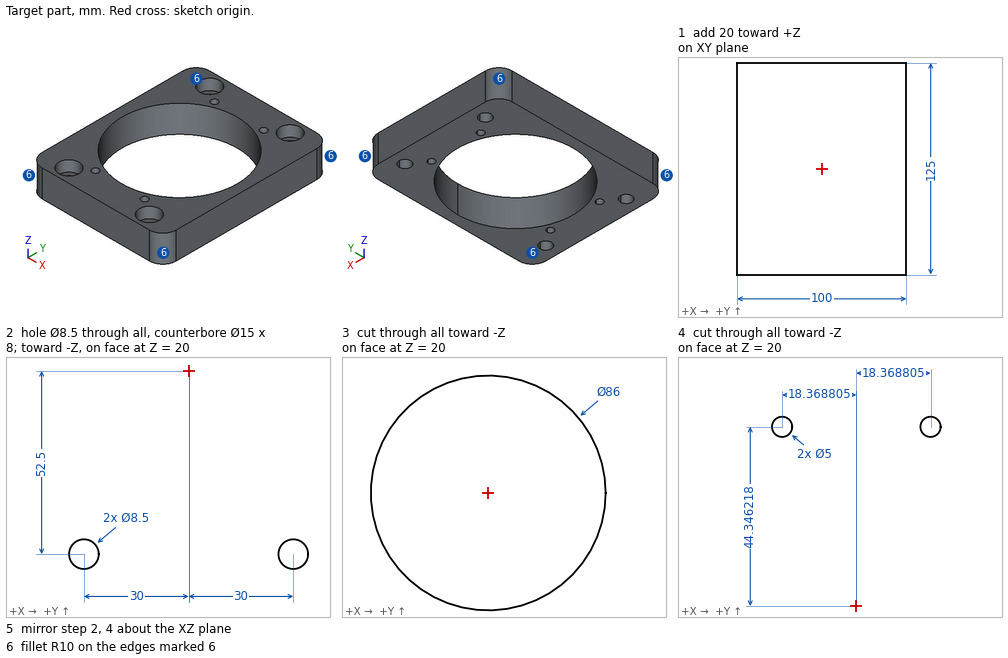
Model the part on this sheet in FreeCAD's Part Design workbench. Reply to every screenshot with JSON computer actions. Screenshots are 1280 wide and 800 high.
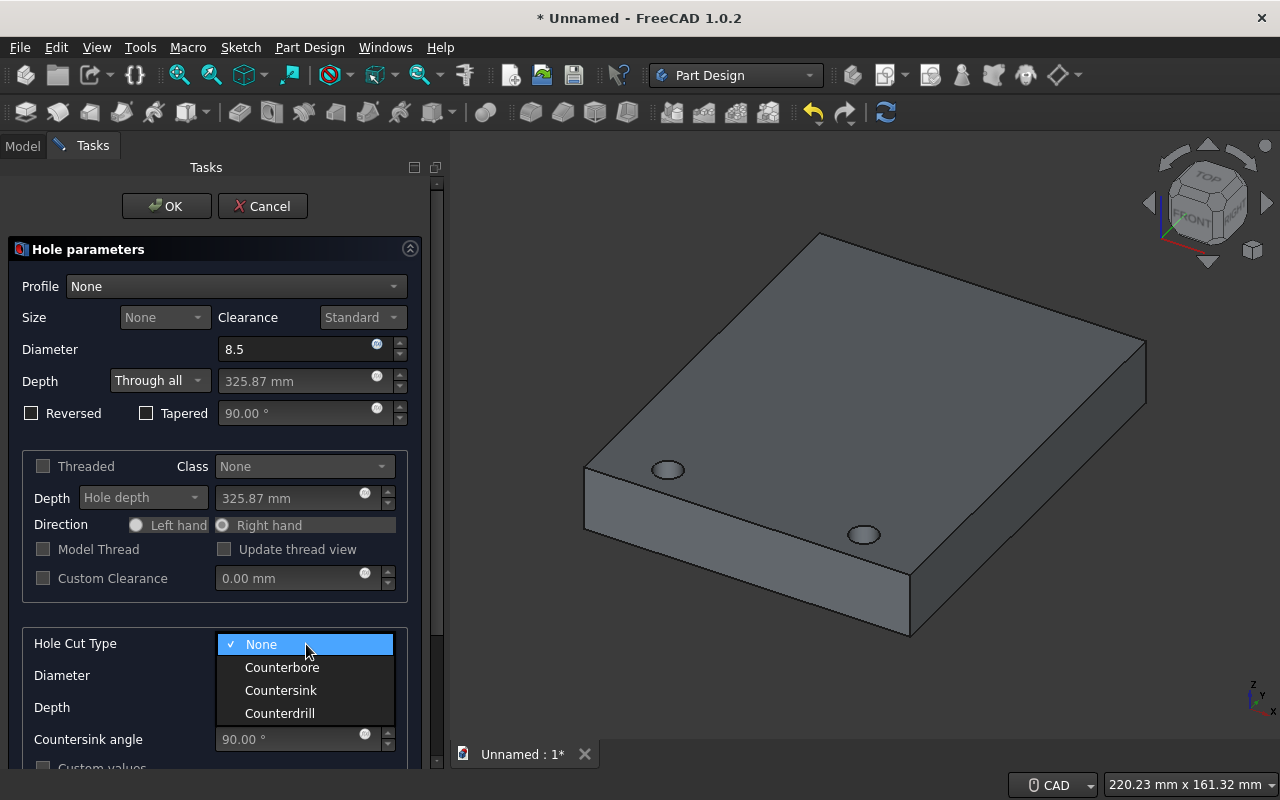
{"action": "left_click", "coordinate": [304, 668]}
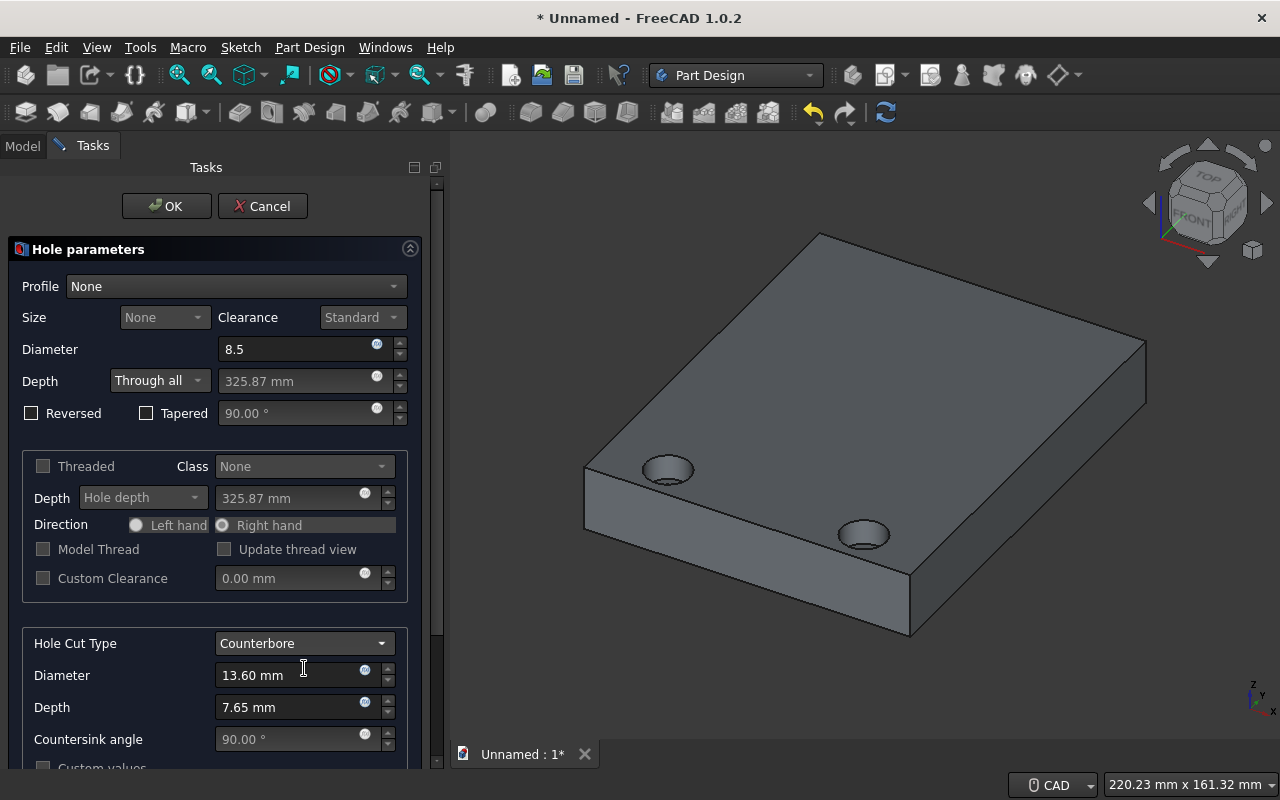
{"action": "triple_click", "coordinate": [298, 675]}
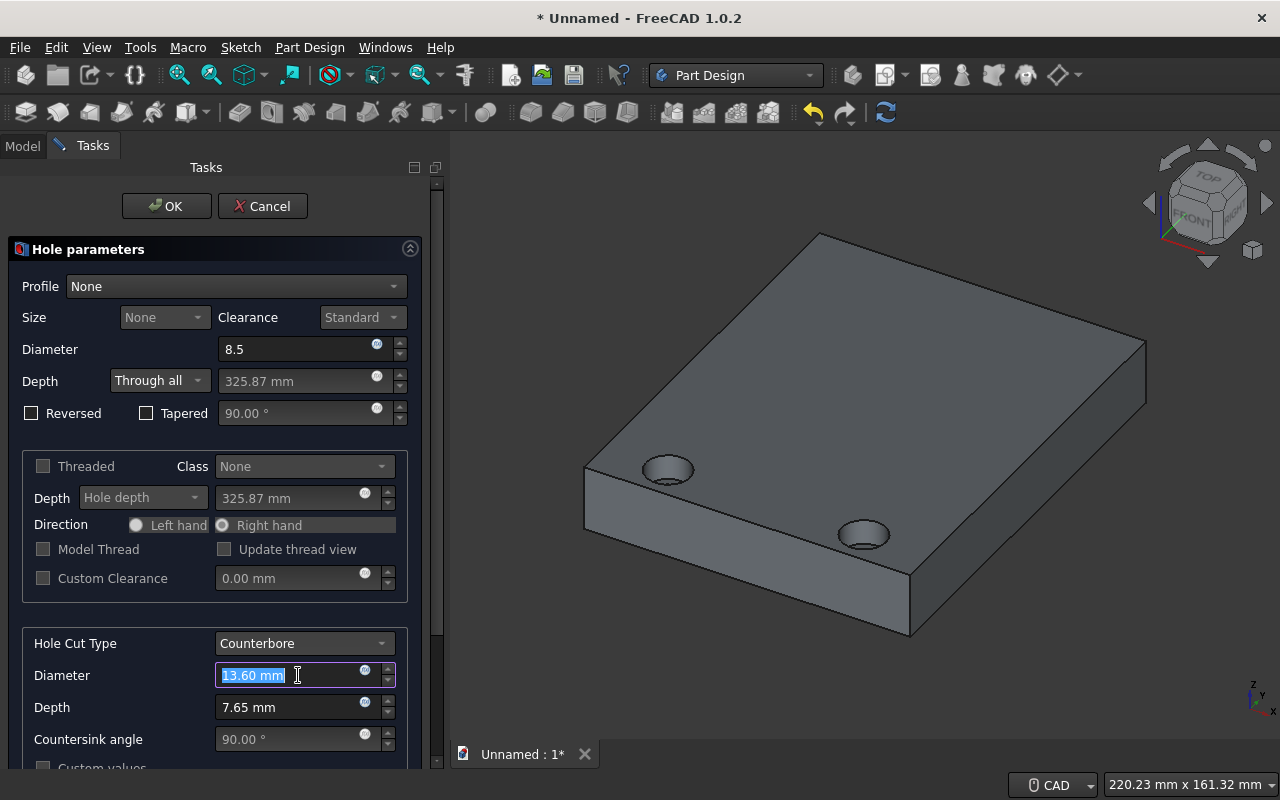
{"action": "type", "text": "15"}
{"action": "key", "text": "Tab"}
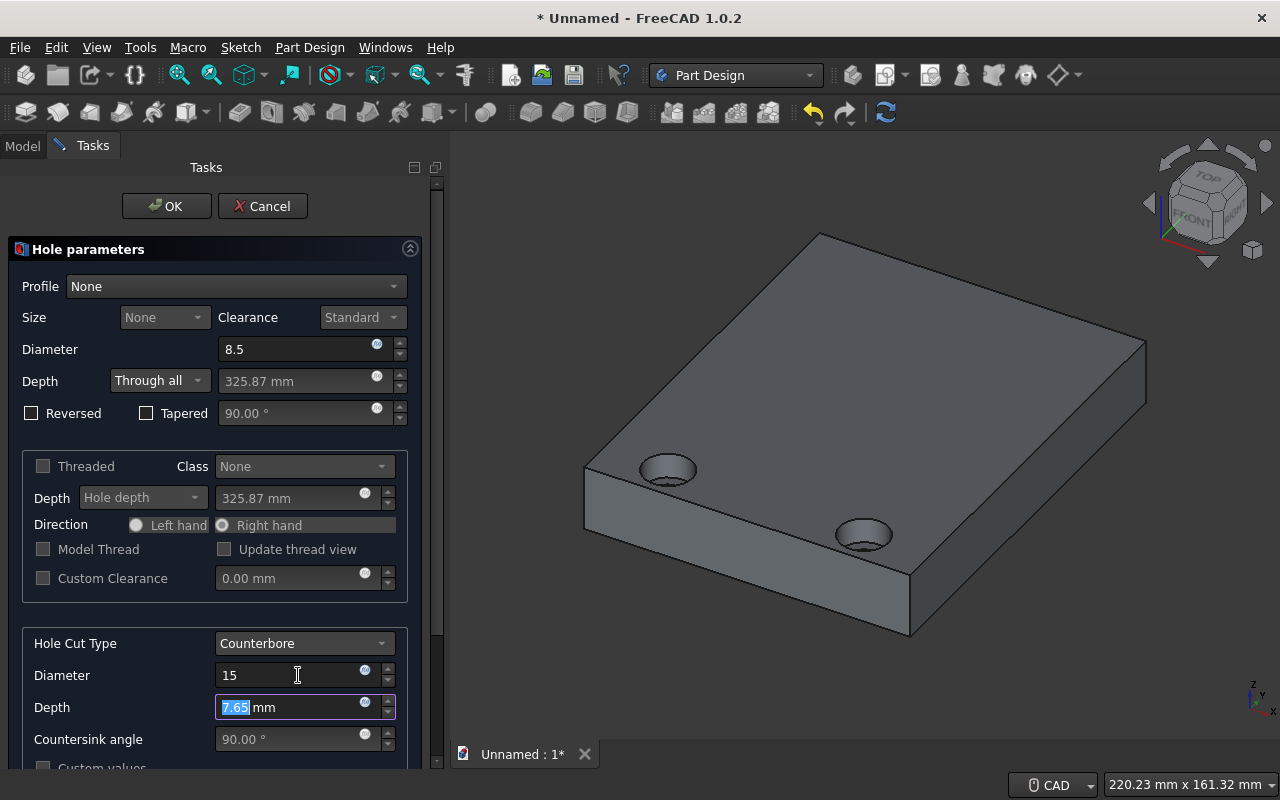
{"action": "type", "text": "8"}
{"action": "key", "text": "Tab"}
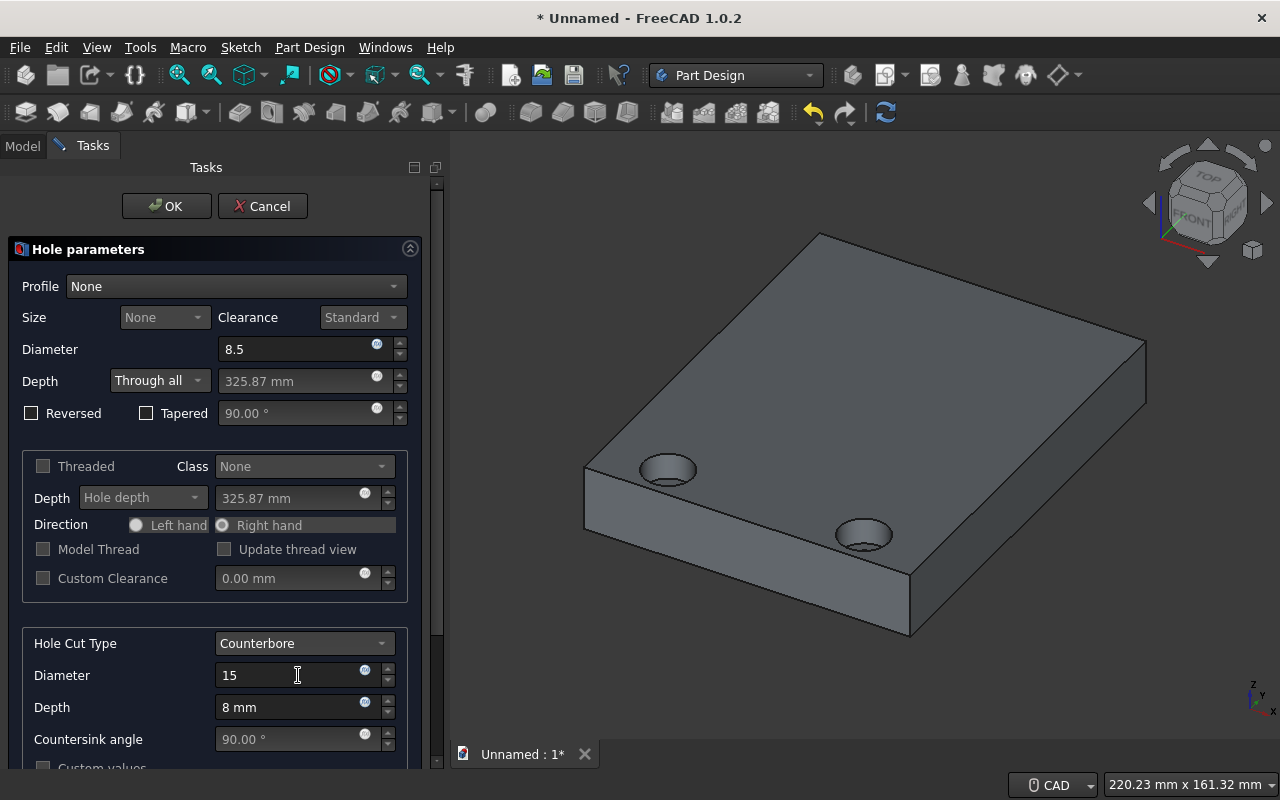
{"action": "left_click", "coordinate": [167, 206]}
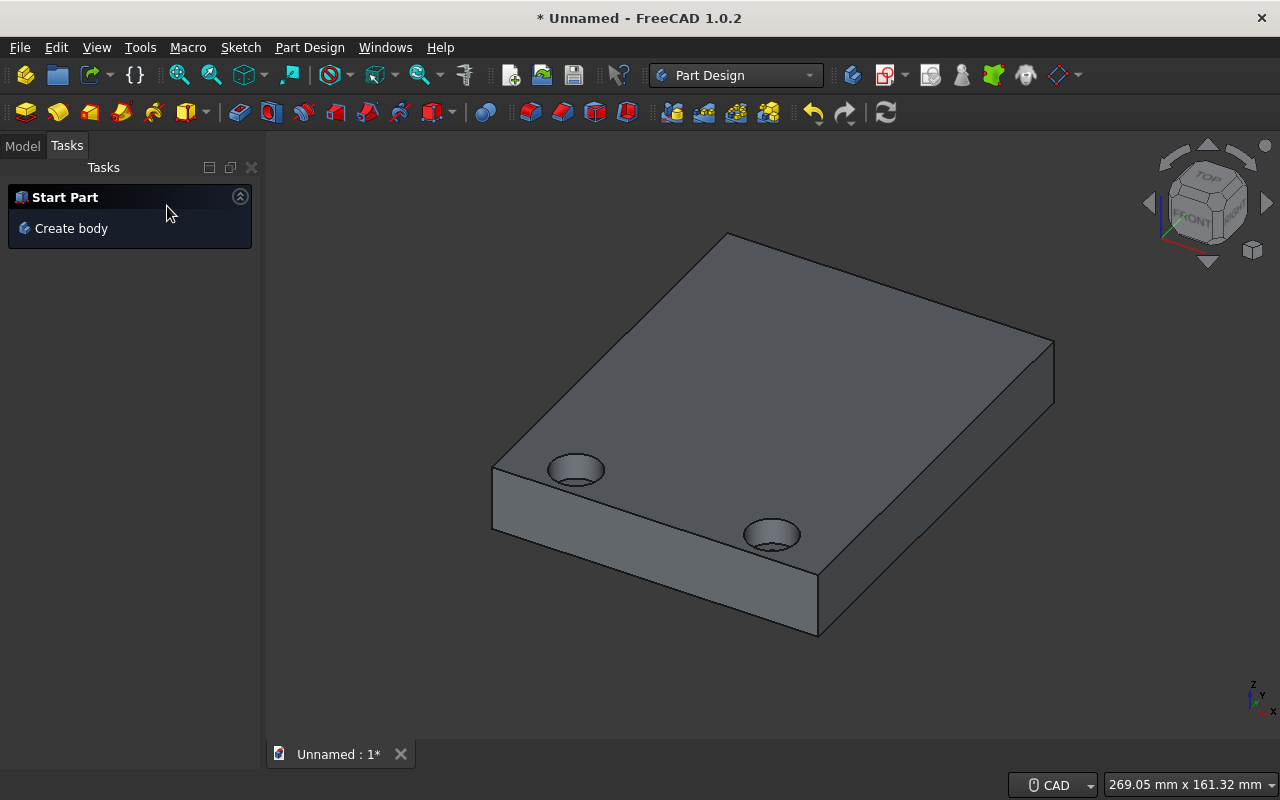
{"action": "left_click", "coordinate": [773, 403]}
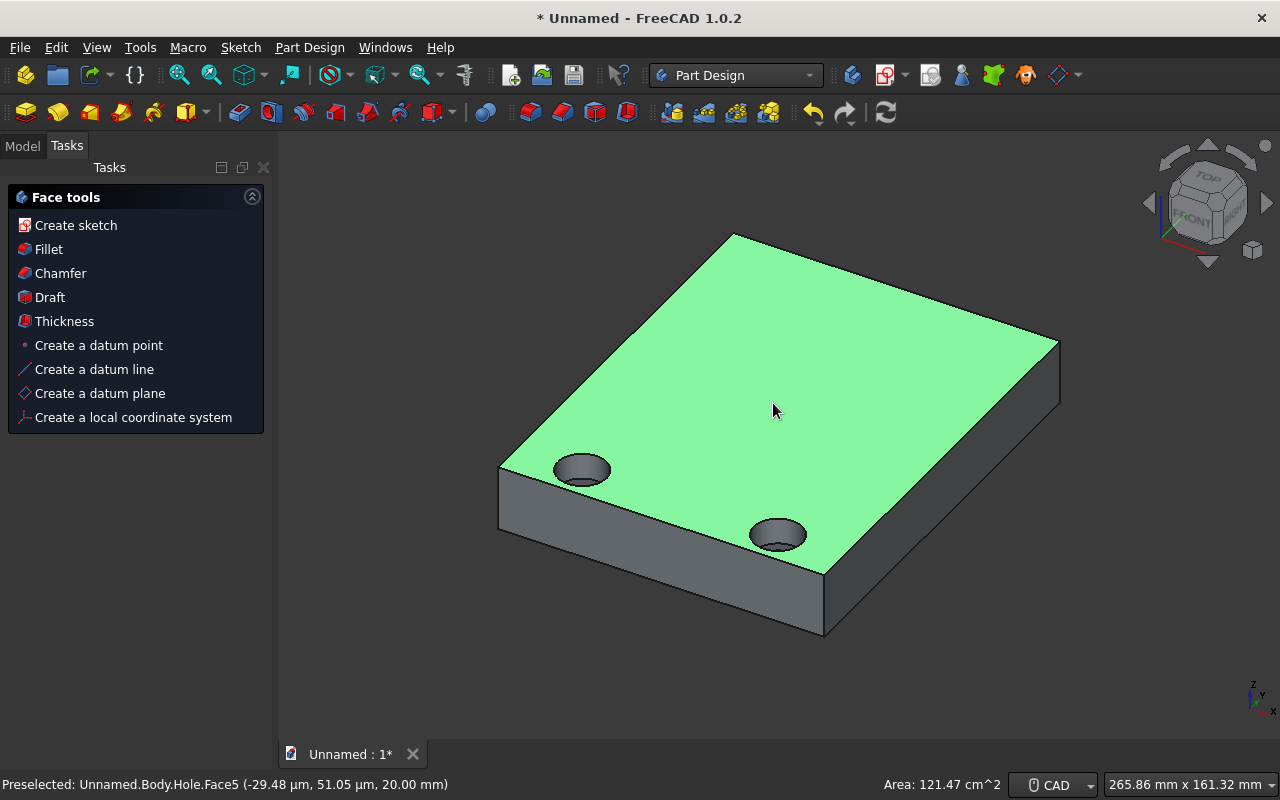
{"action": "left_click", "coordinate": [886, 76]}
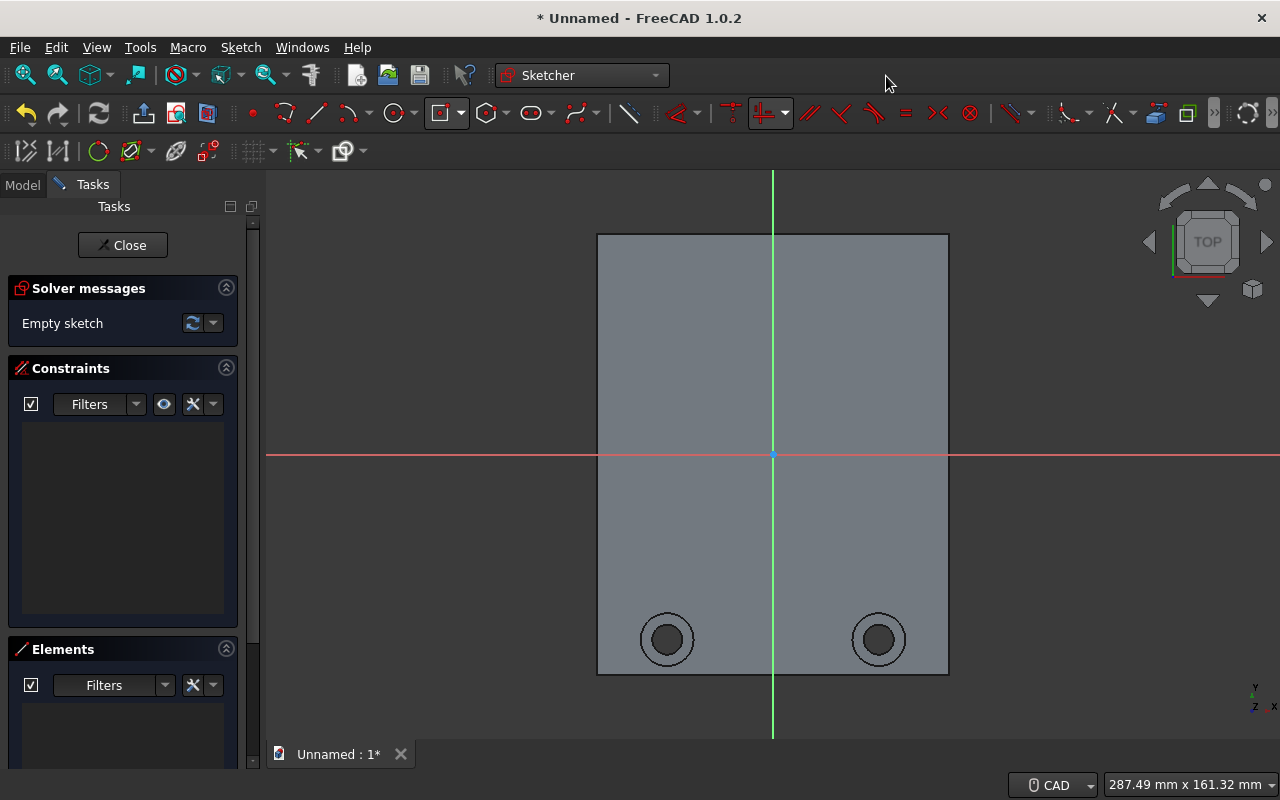
{"action": "left_click", "coordinate": [394, 114]}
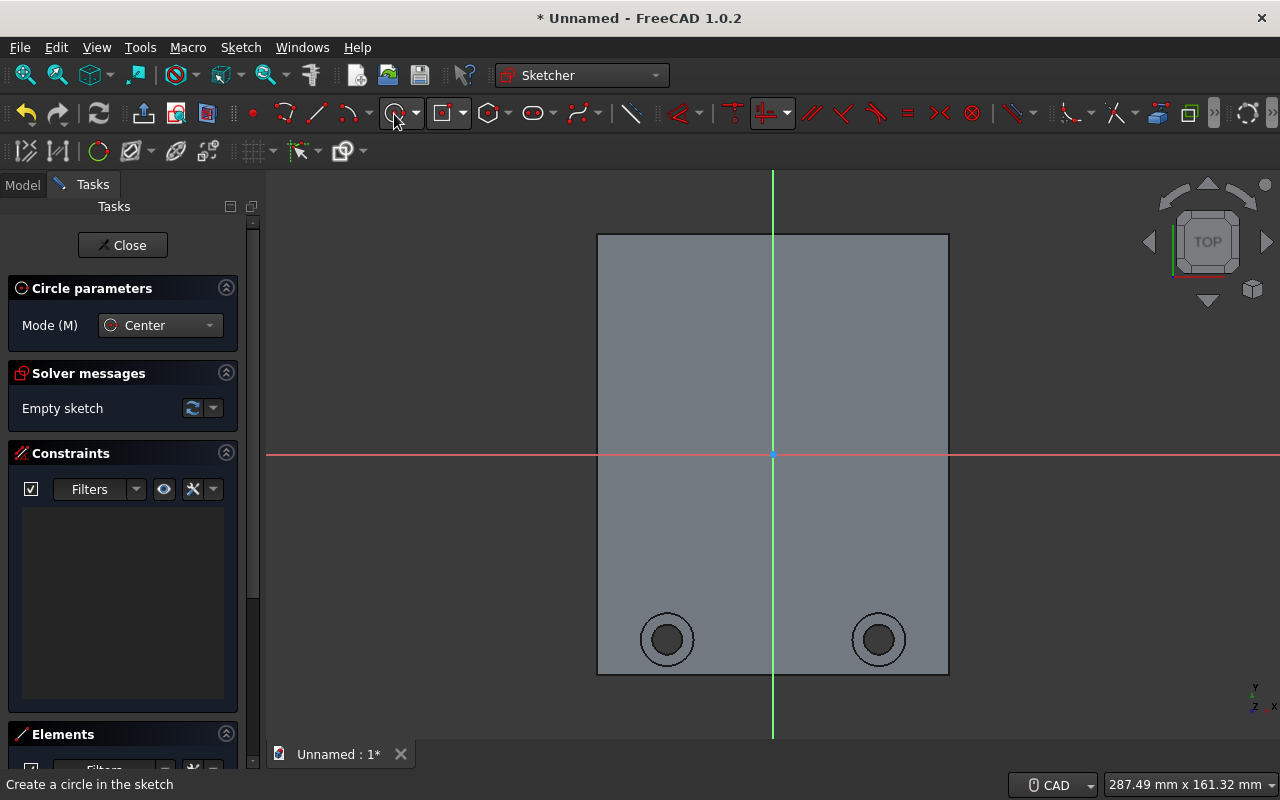
{"action": "left_click", "coordinate": [773, 454]}
{"action": "mouse_move", "coordinate": [880, 347]}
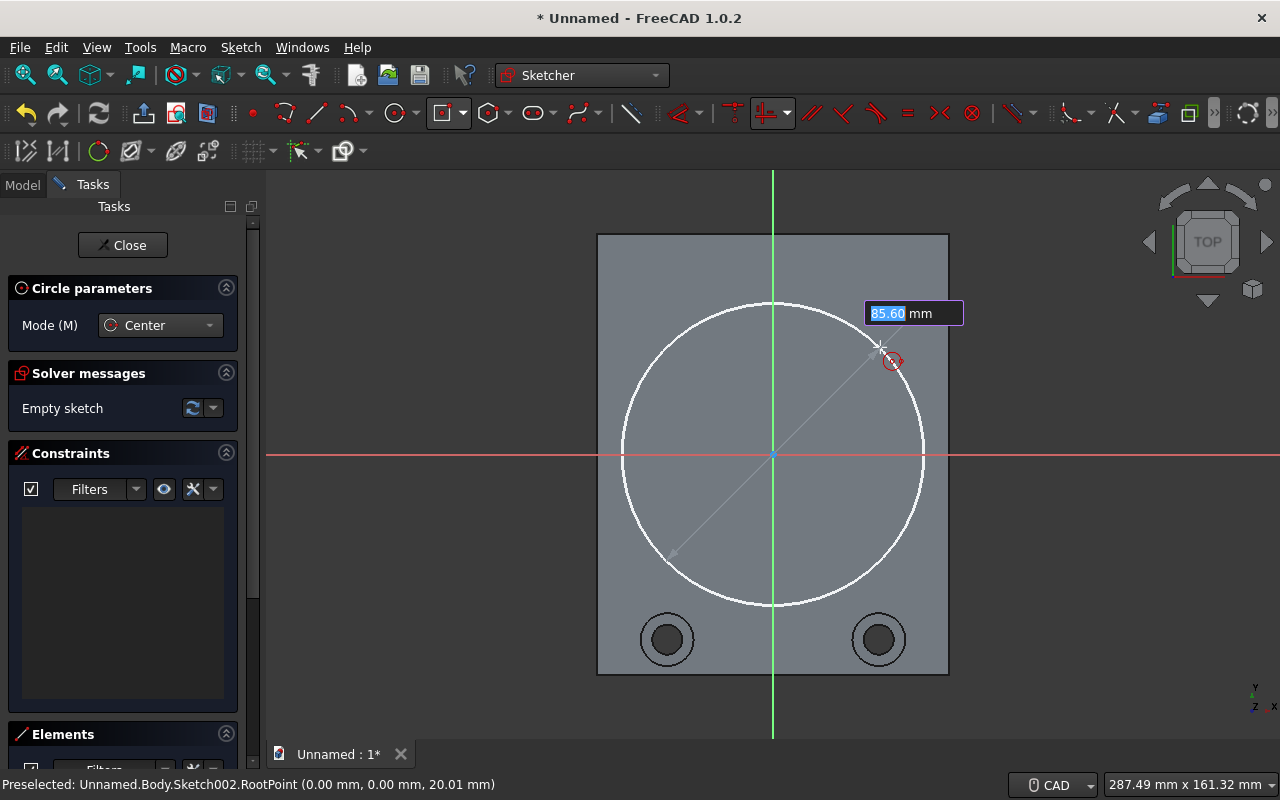
{"action": "type", "text": "86"}
{"action": "key", "text": "Return"}
{"action": "key", "text": "Escape"}